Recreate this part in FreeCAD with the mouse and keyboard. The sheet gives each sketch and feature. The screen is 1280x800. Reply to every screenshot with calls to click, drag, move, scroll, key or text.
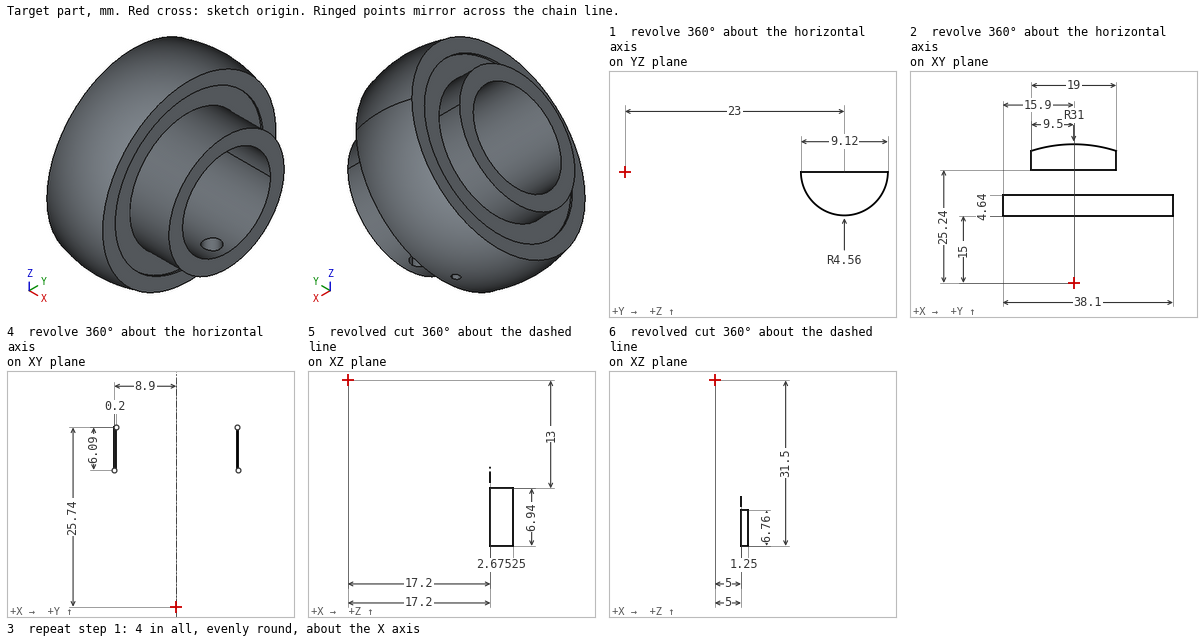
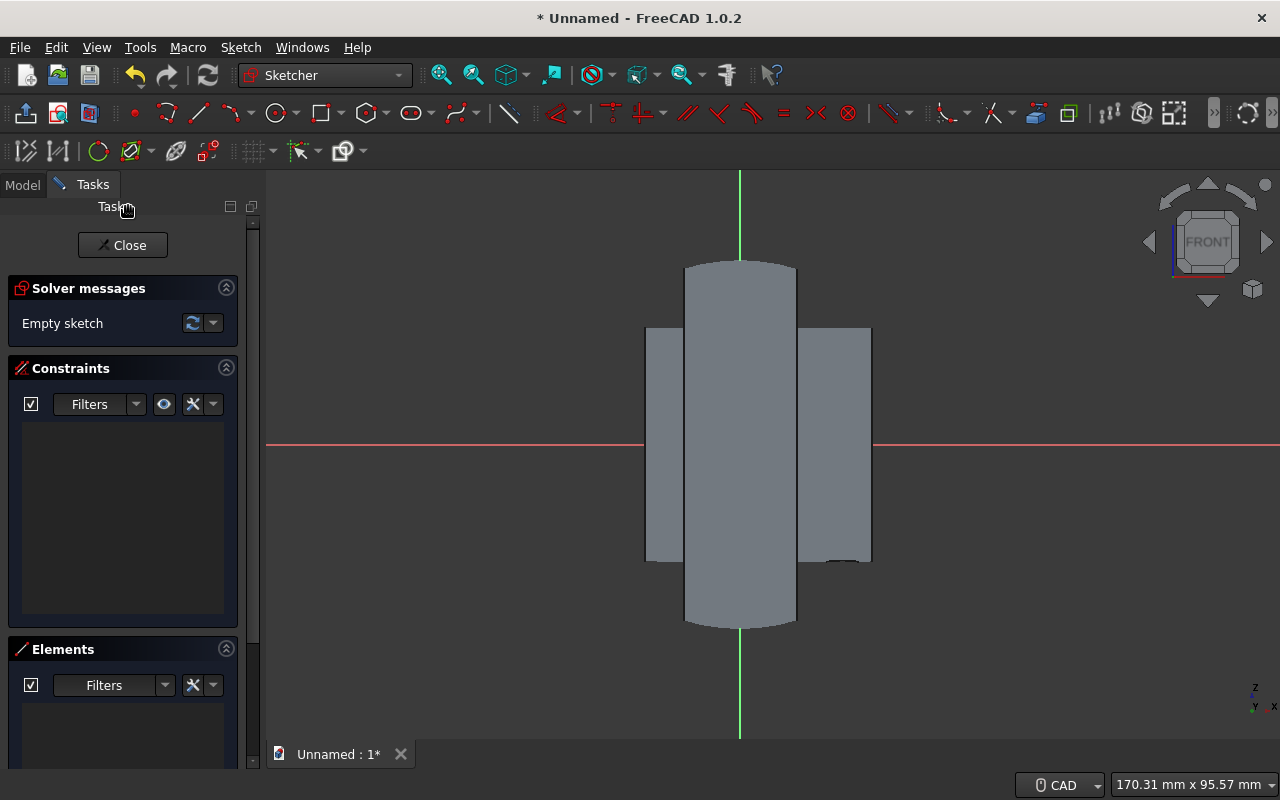
click(90, 114)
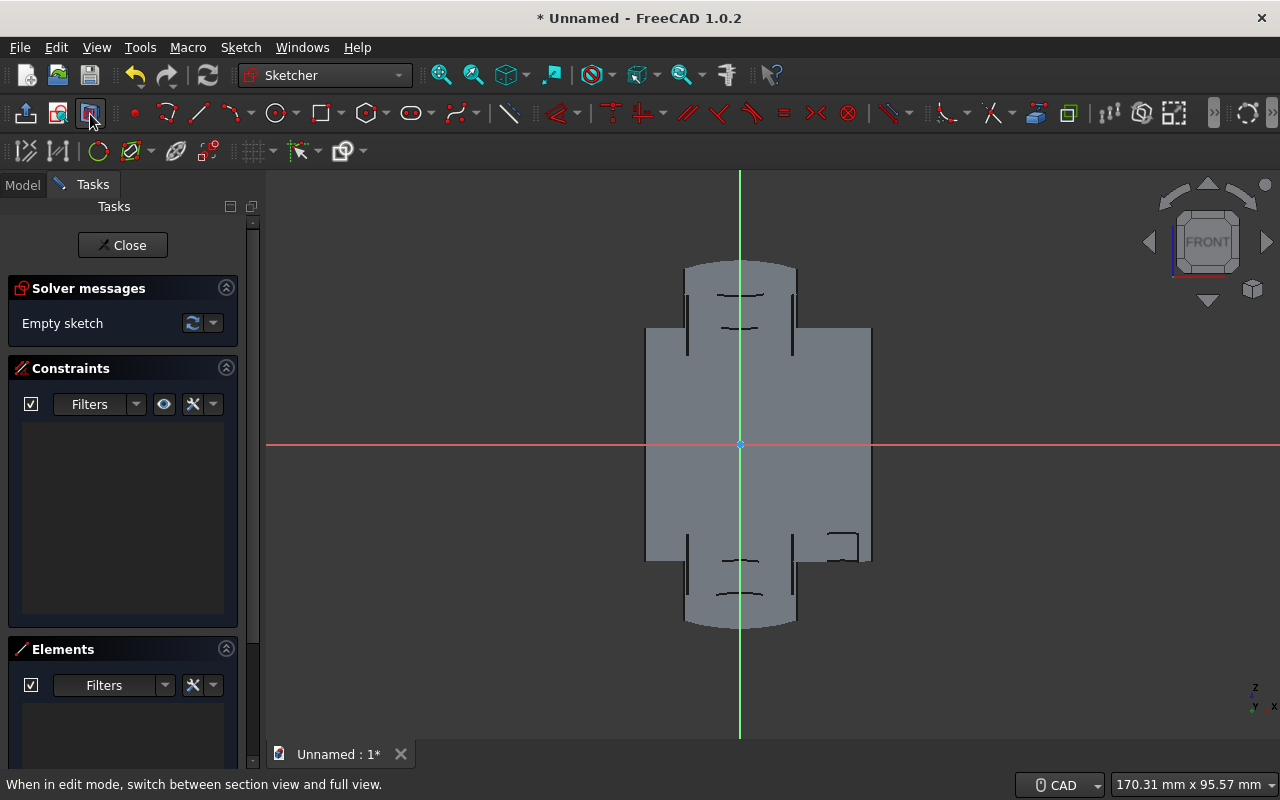
scroll(787, 634, up, 9)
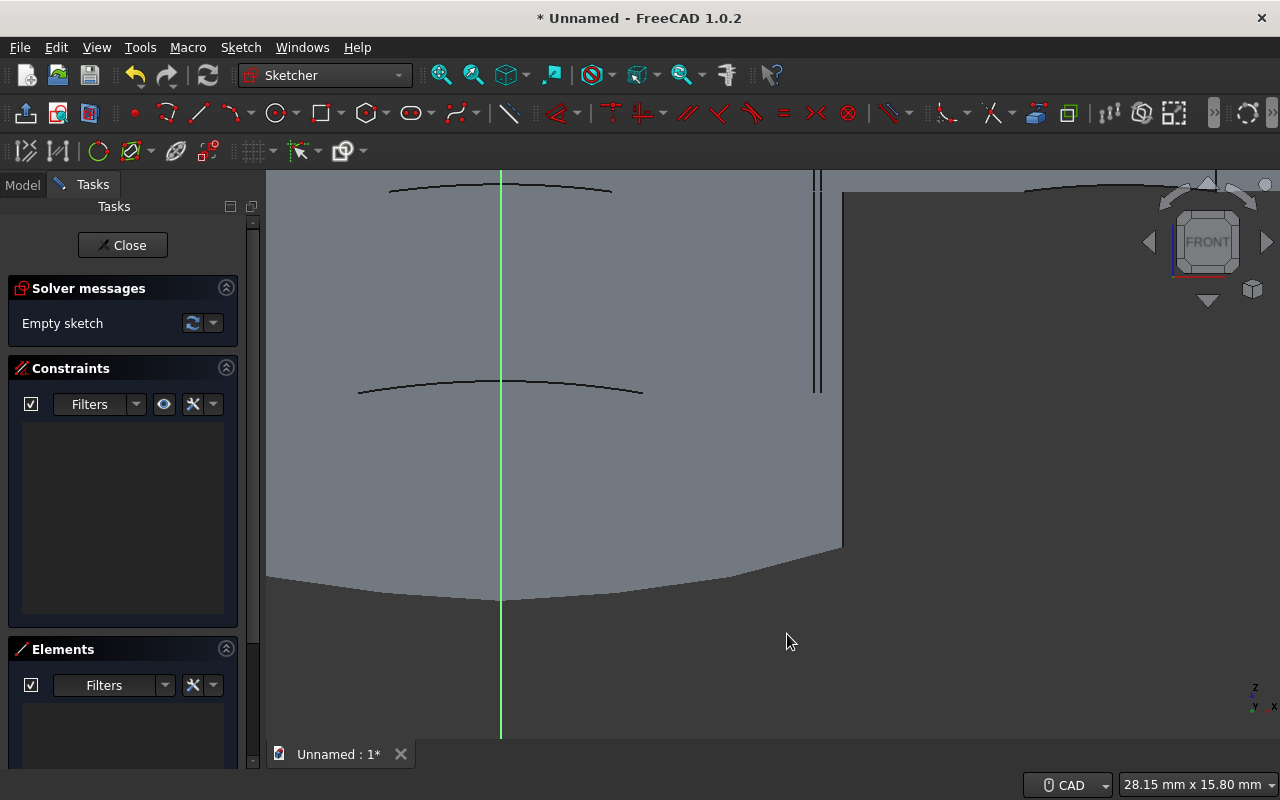
click(322, 114)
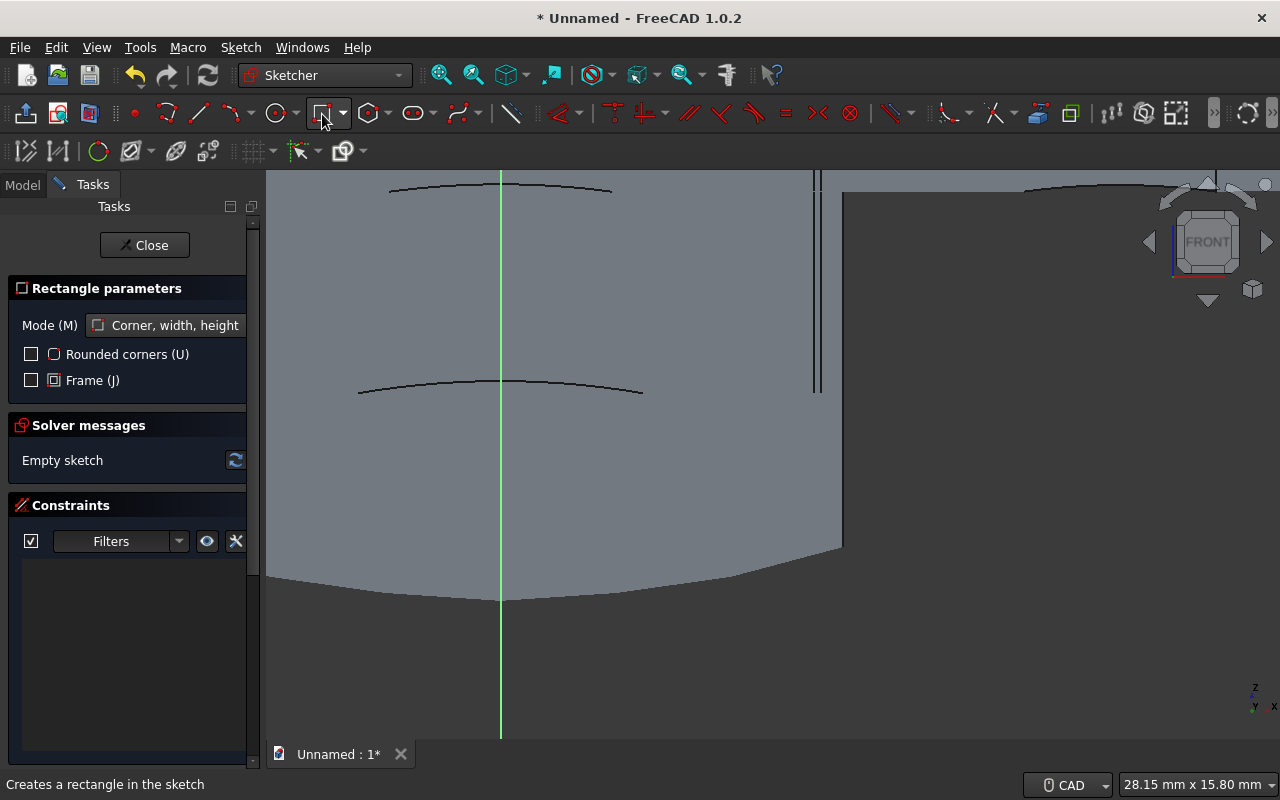
click(681, 375)
click(726, 619)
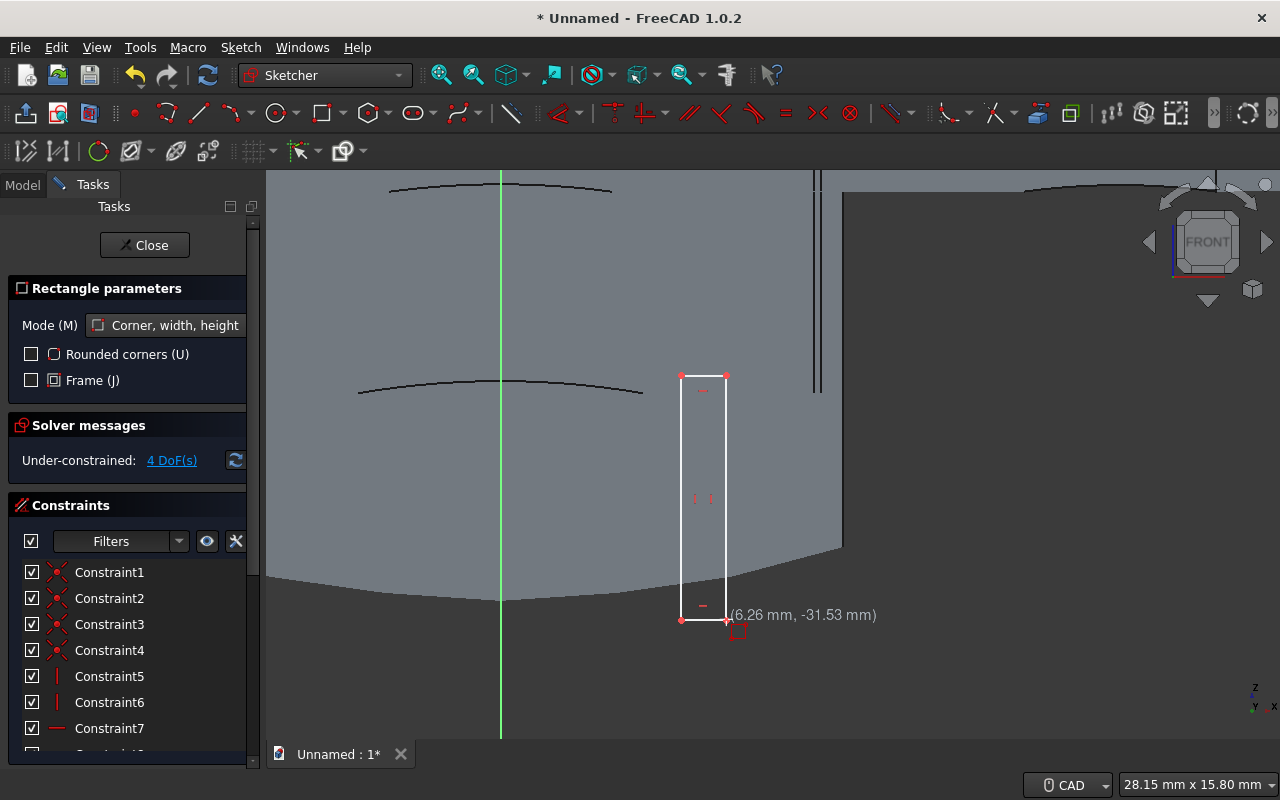
click(200, 114)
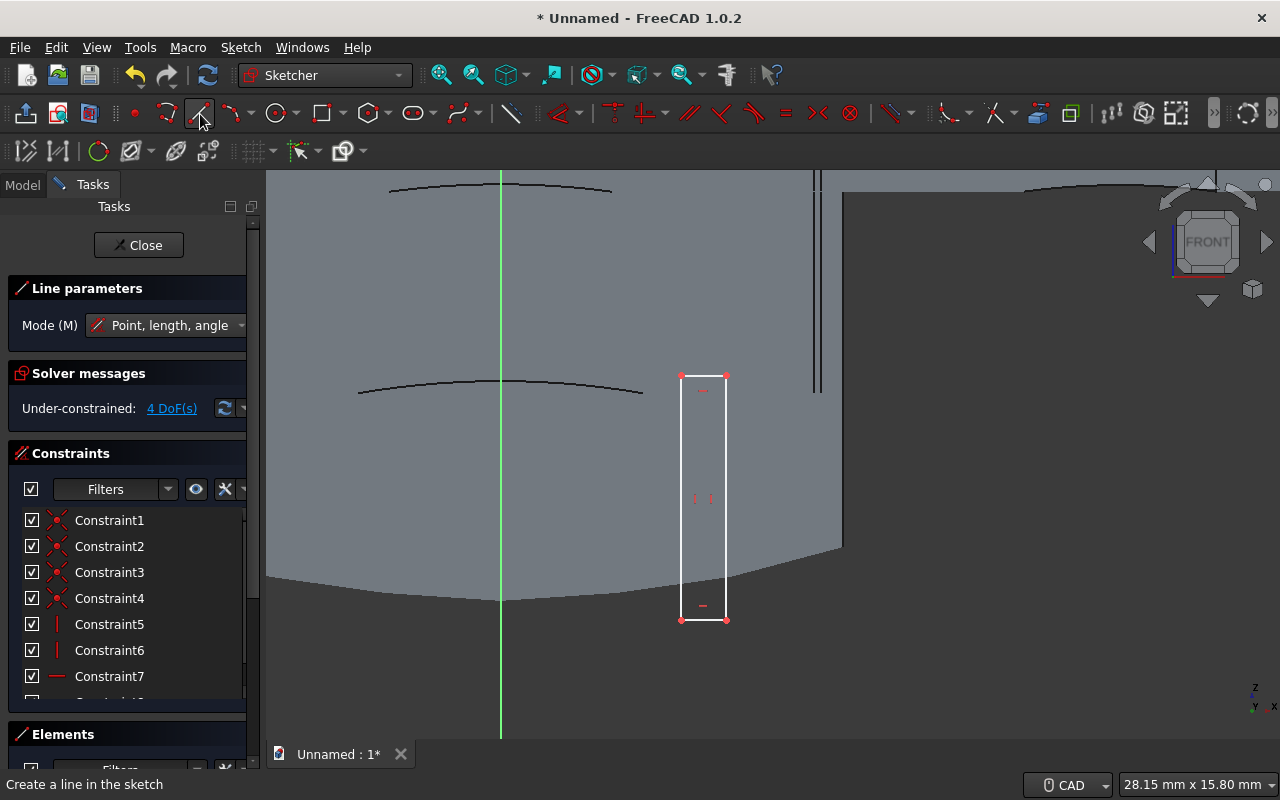
click(681, 351)
click(681, 278)
key(Escape)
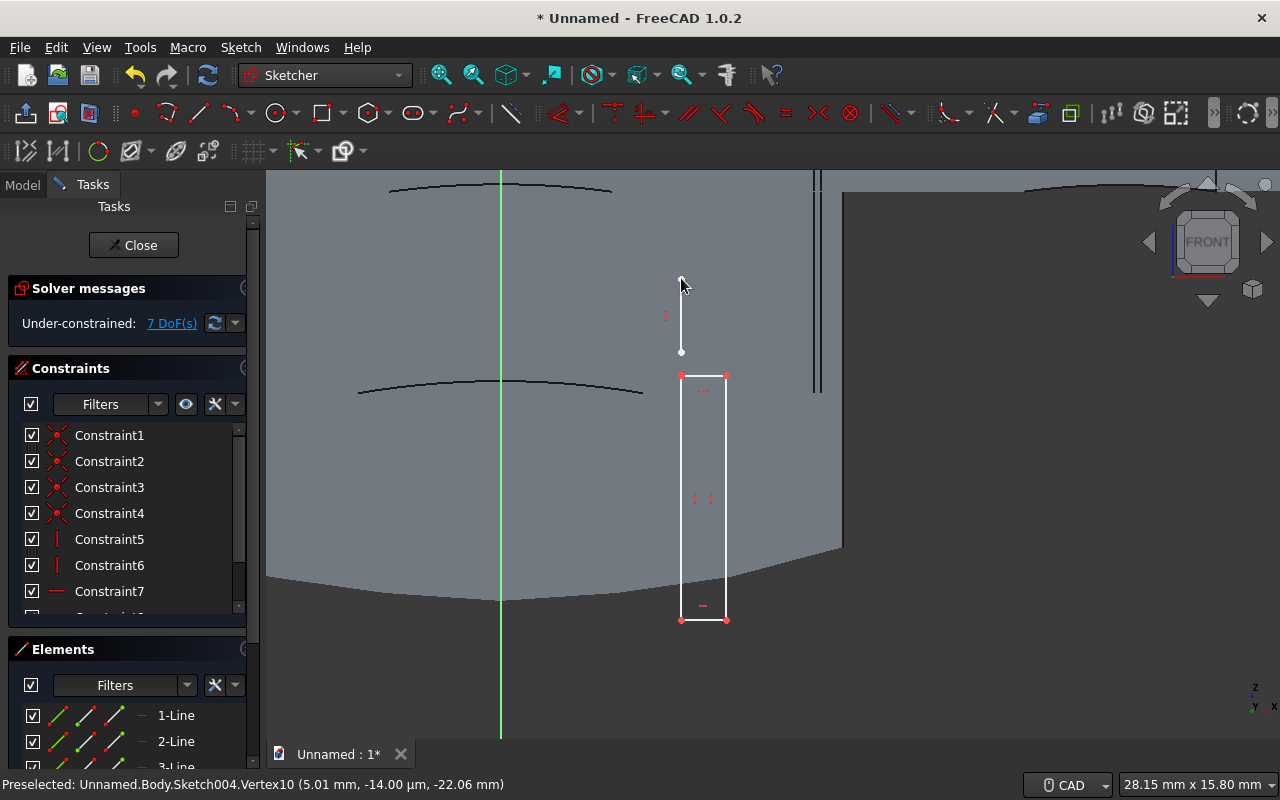
click(681, 330)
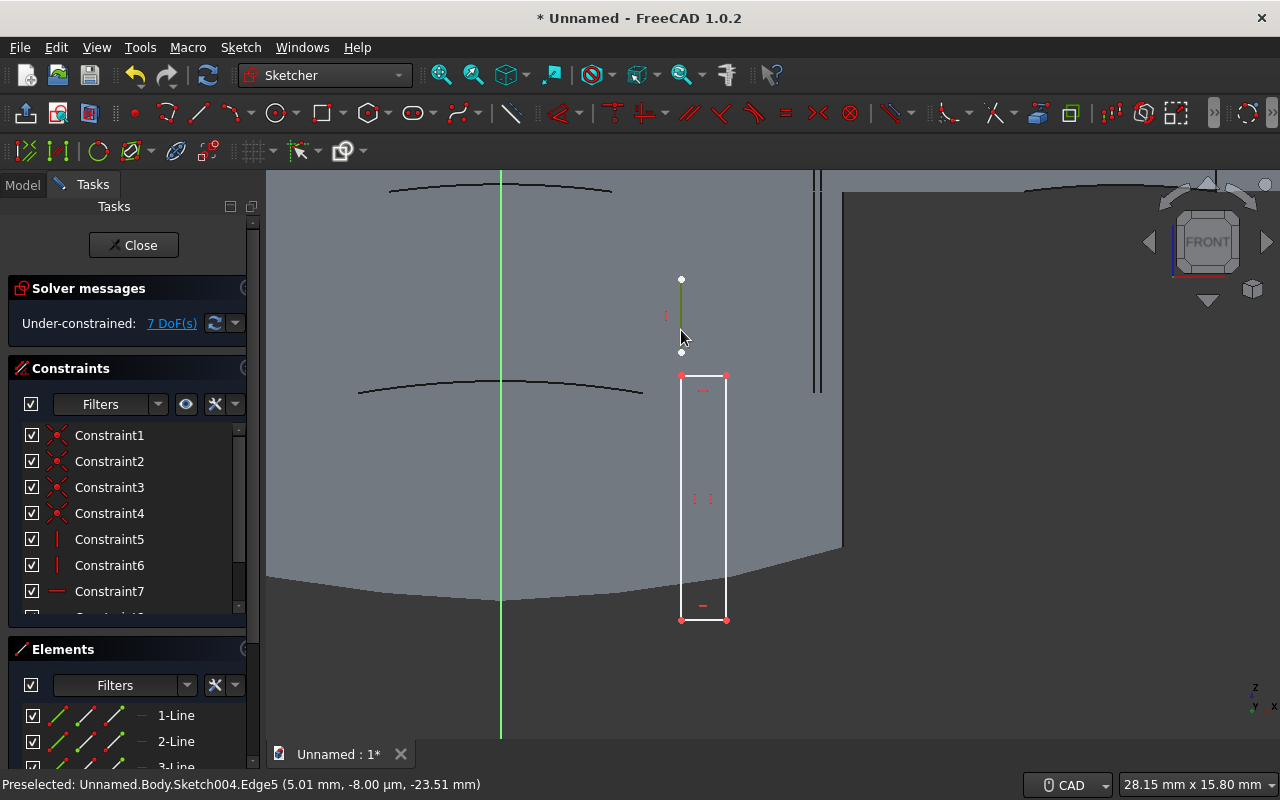
click(512, 114)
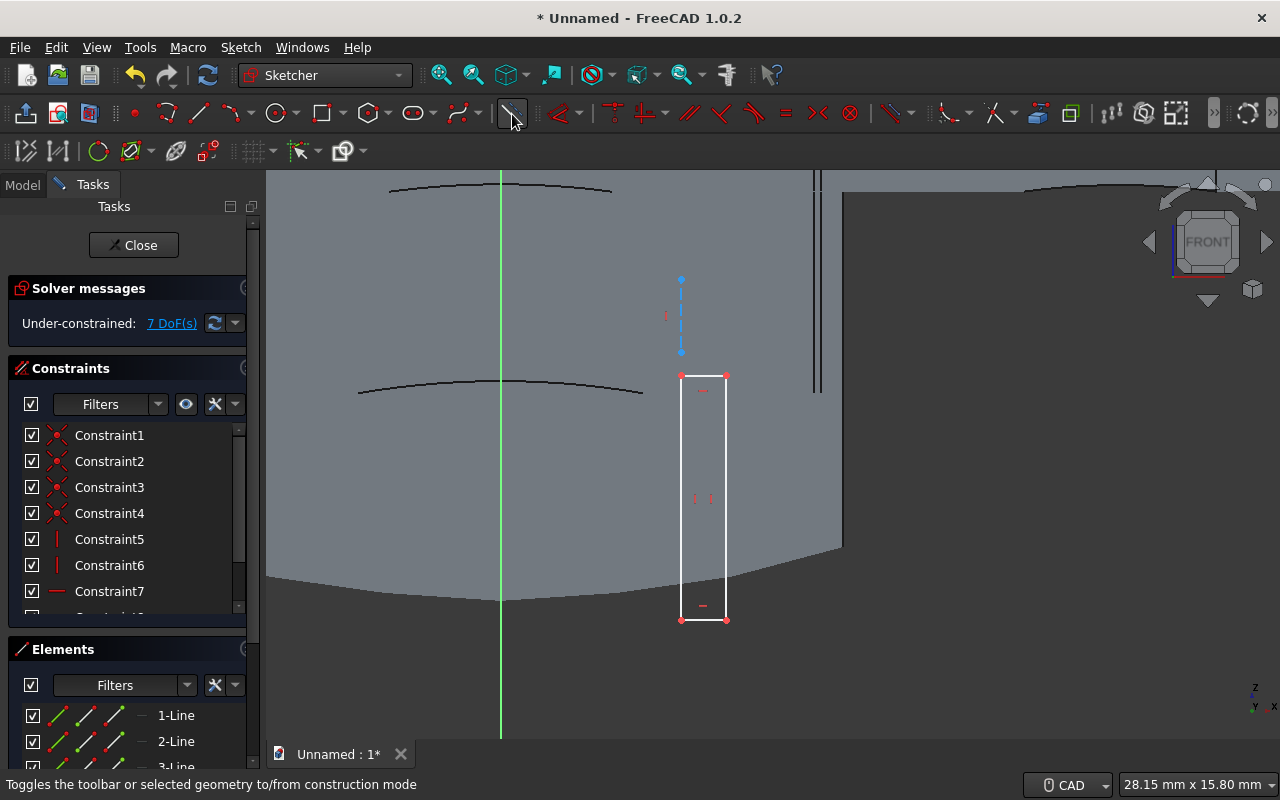
click(558, 114)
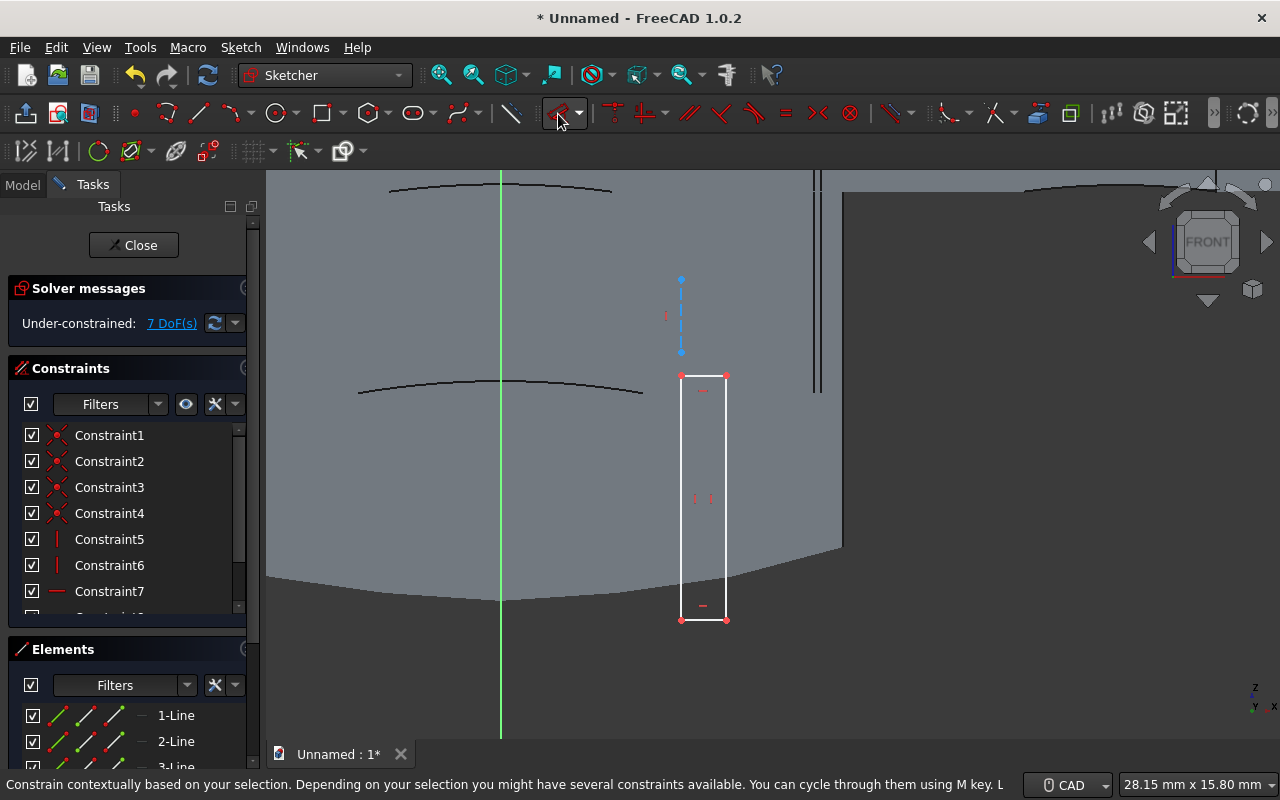
click(681, 376)
click(591, 410)